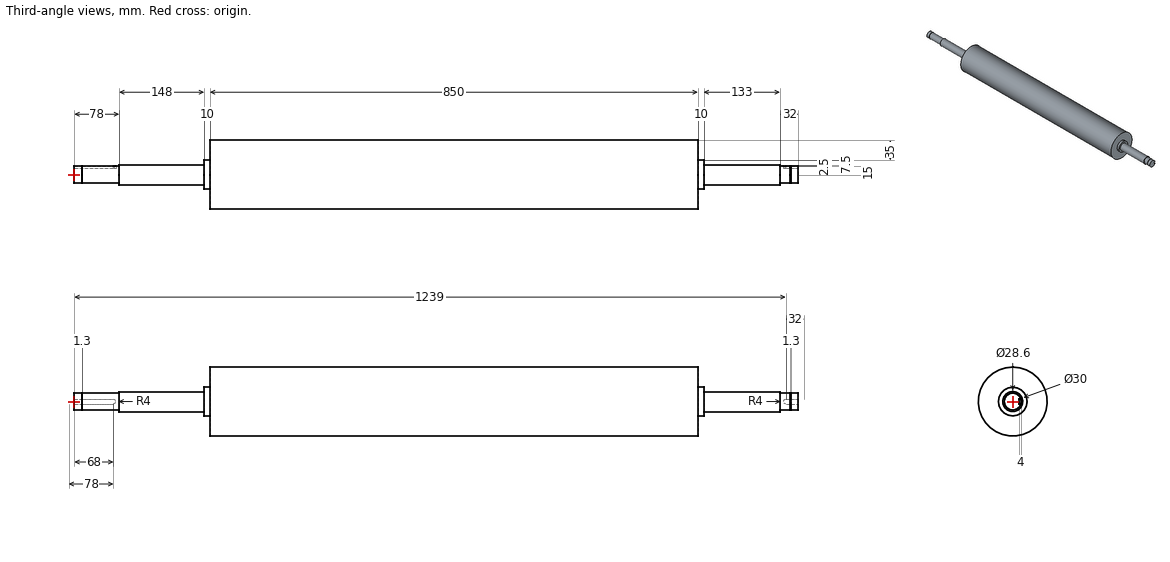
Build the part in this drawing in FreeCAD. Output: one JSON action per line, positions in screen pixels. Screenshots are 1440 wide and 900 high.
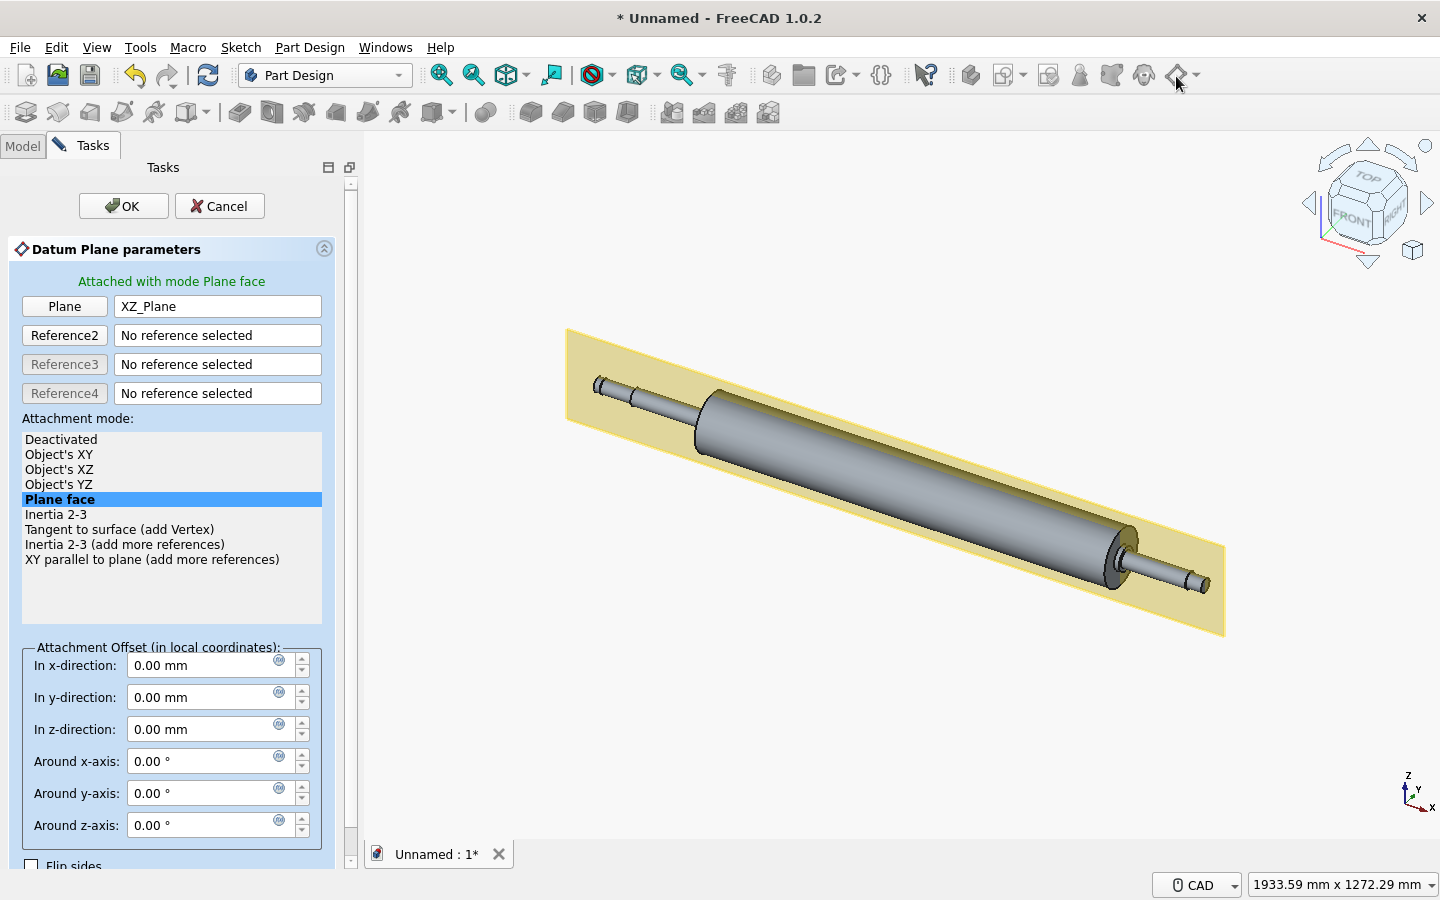
{"action": "triple_click", "coordinate": [210, 729]}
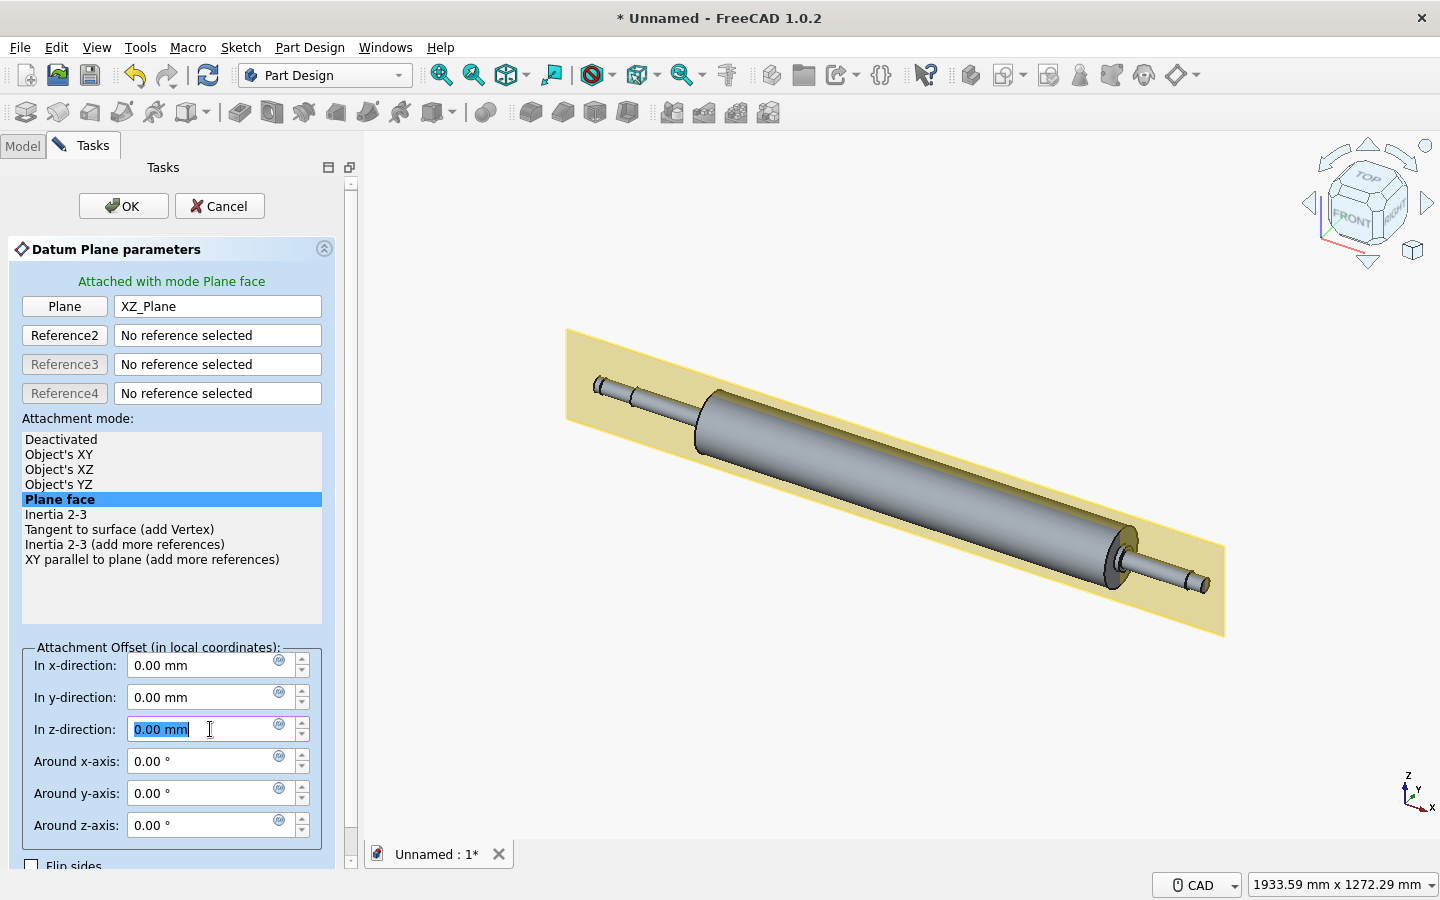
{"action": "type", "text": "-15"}
{"action": "key", "text": "Tab"}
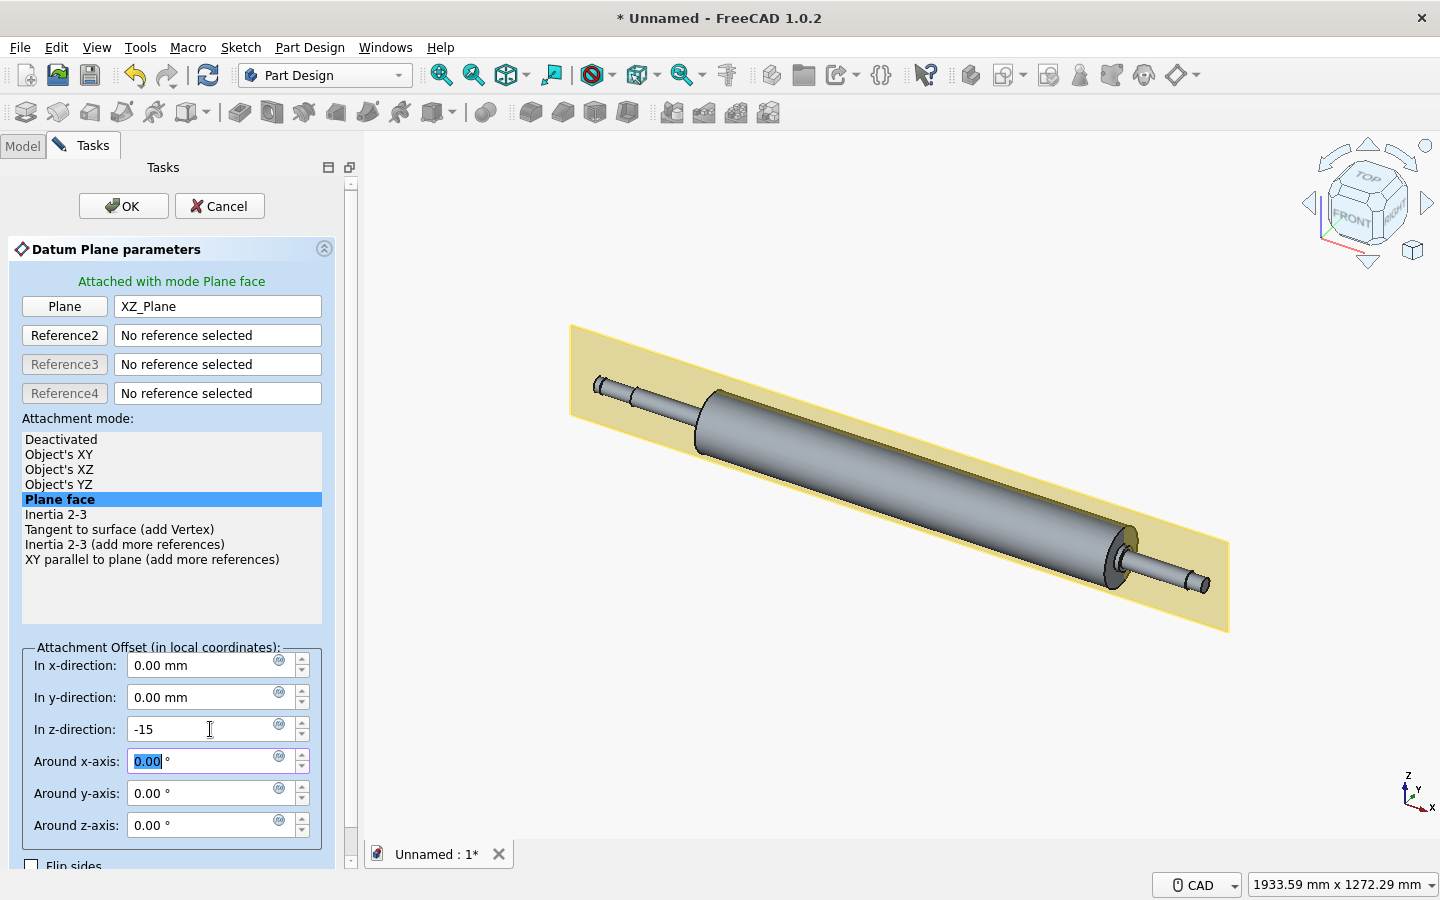
{"action": "left_click", "coordinate": [124, 206]}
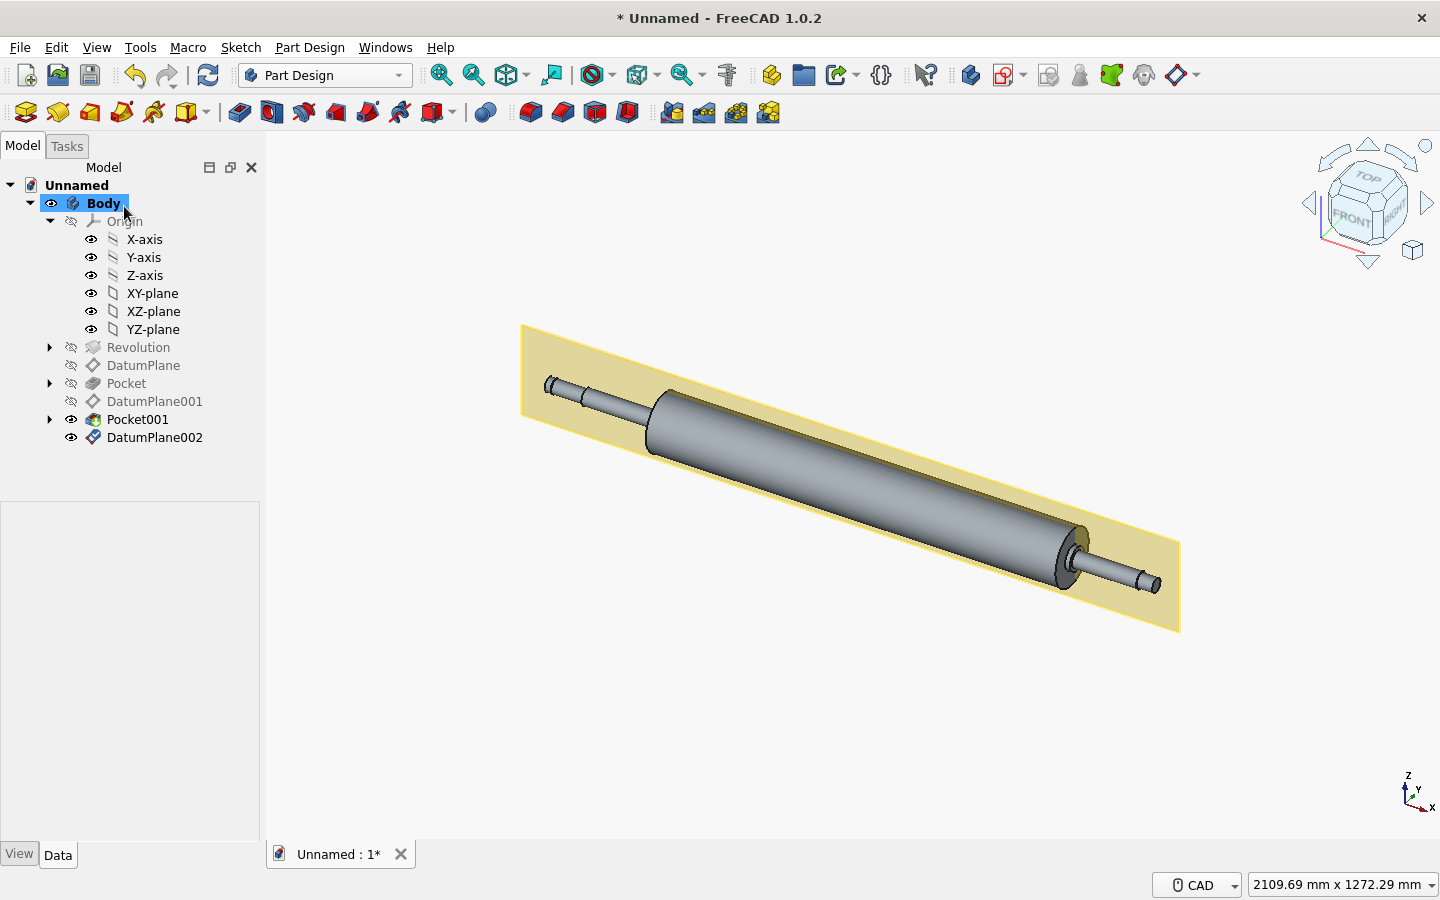
{"action": "left_click", "coordinate": [116, 437]}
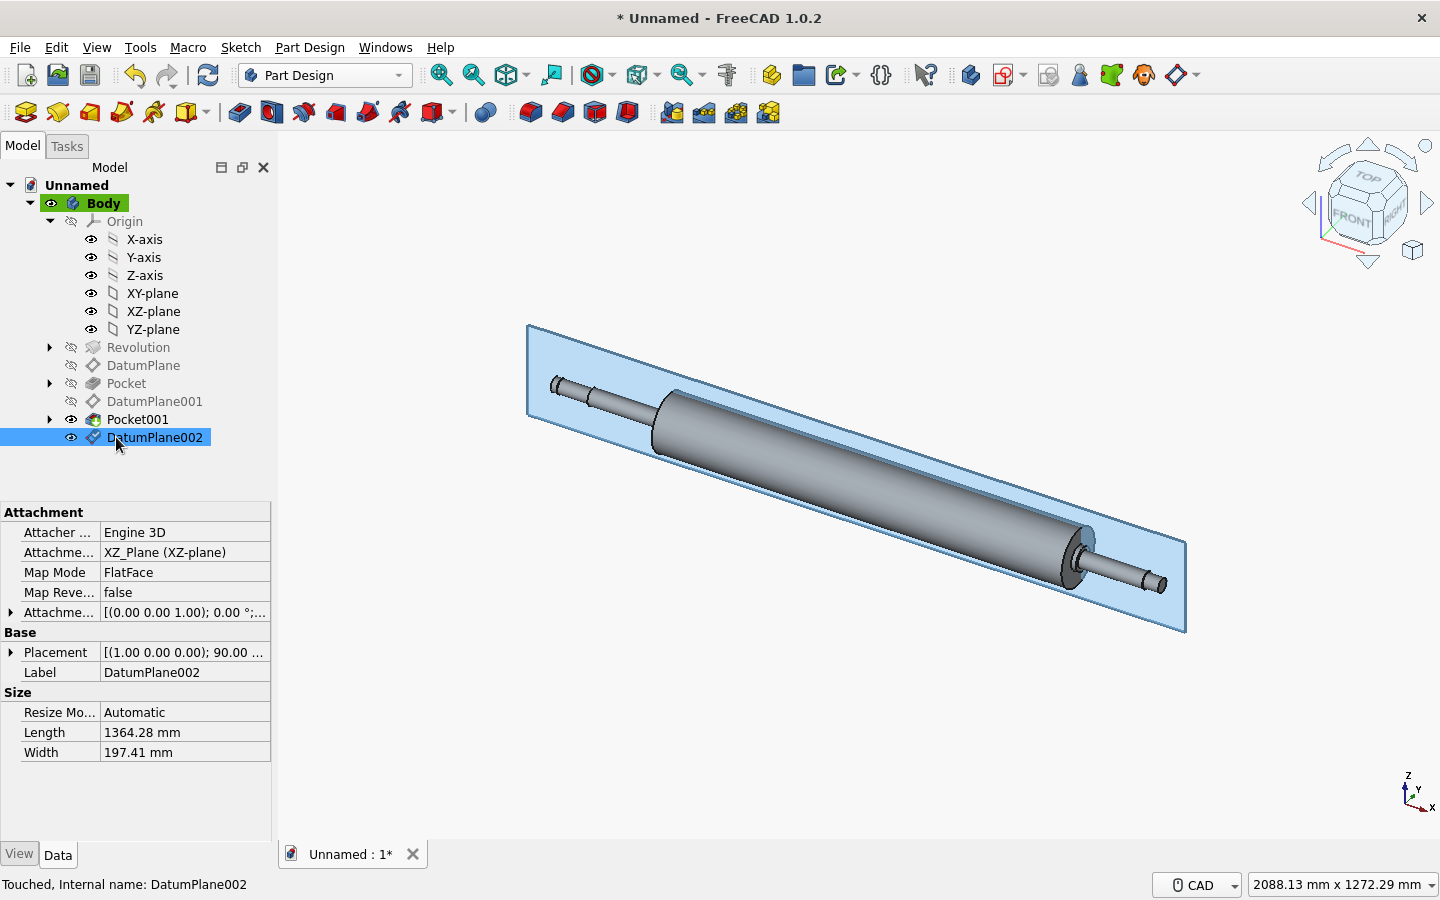
{"action": "left_click", "coordinate": [1004, 76]}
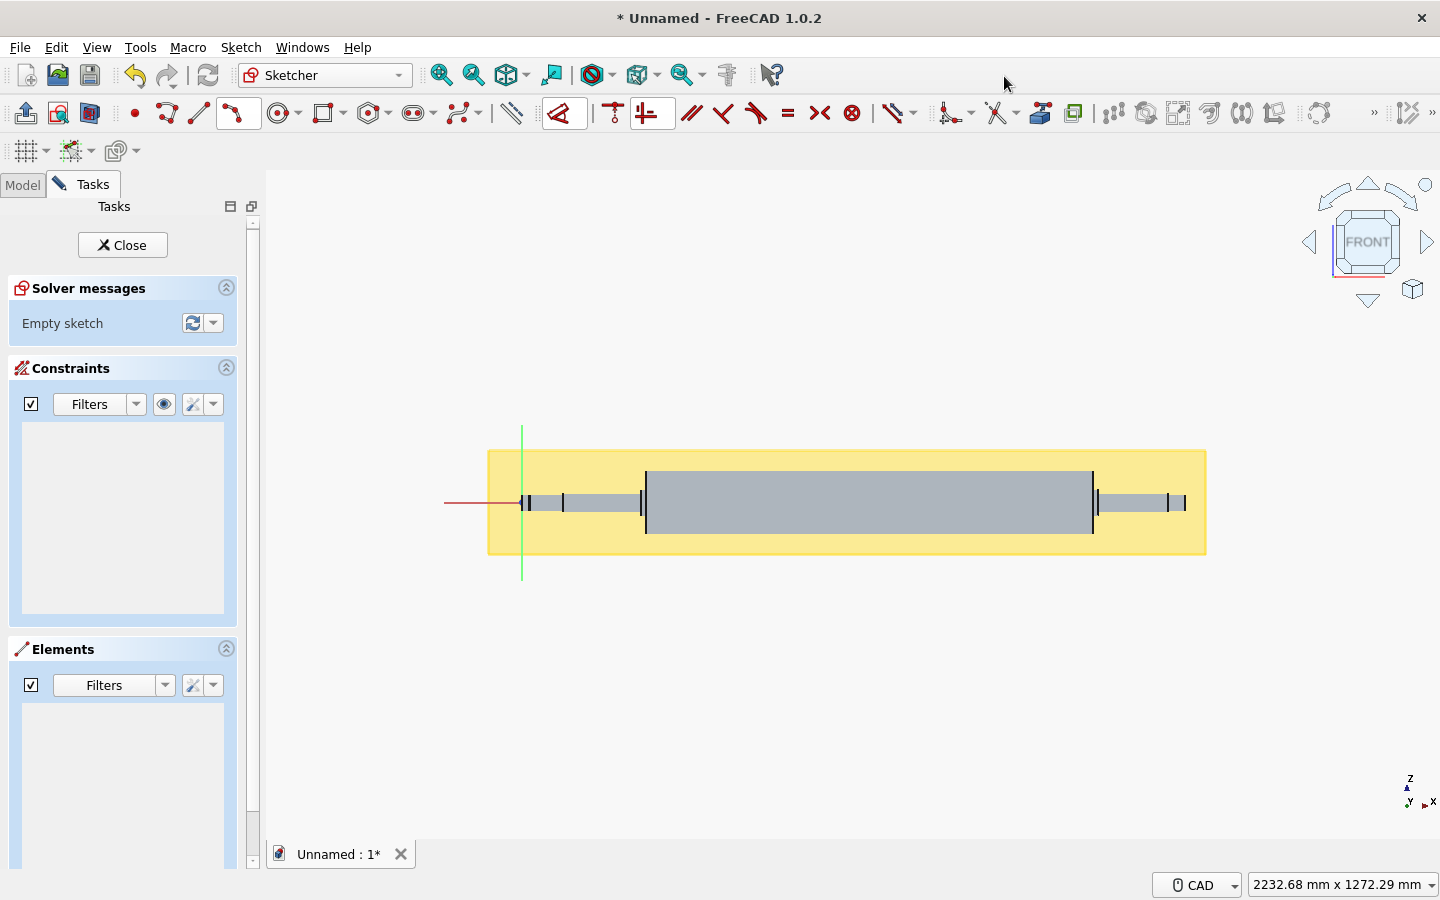
{"action": "key", "text": "q s"}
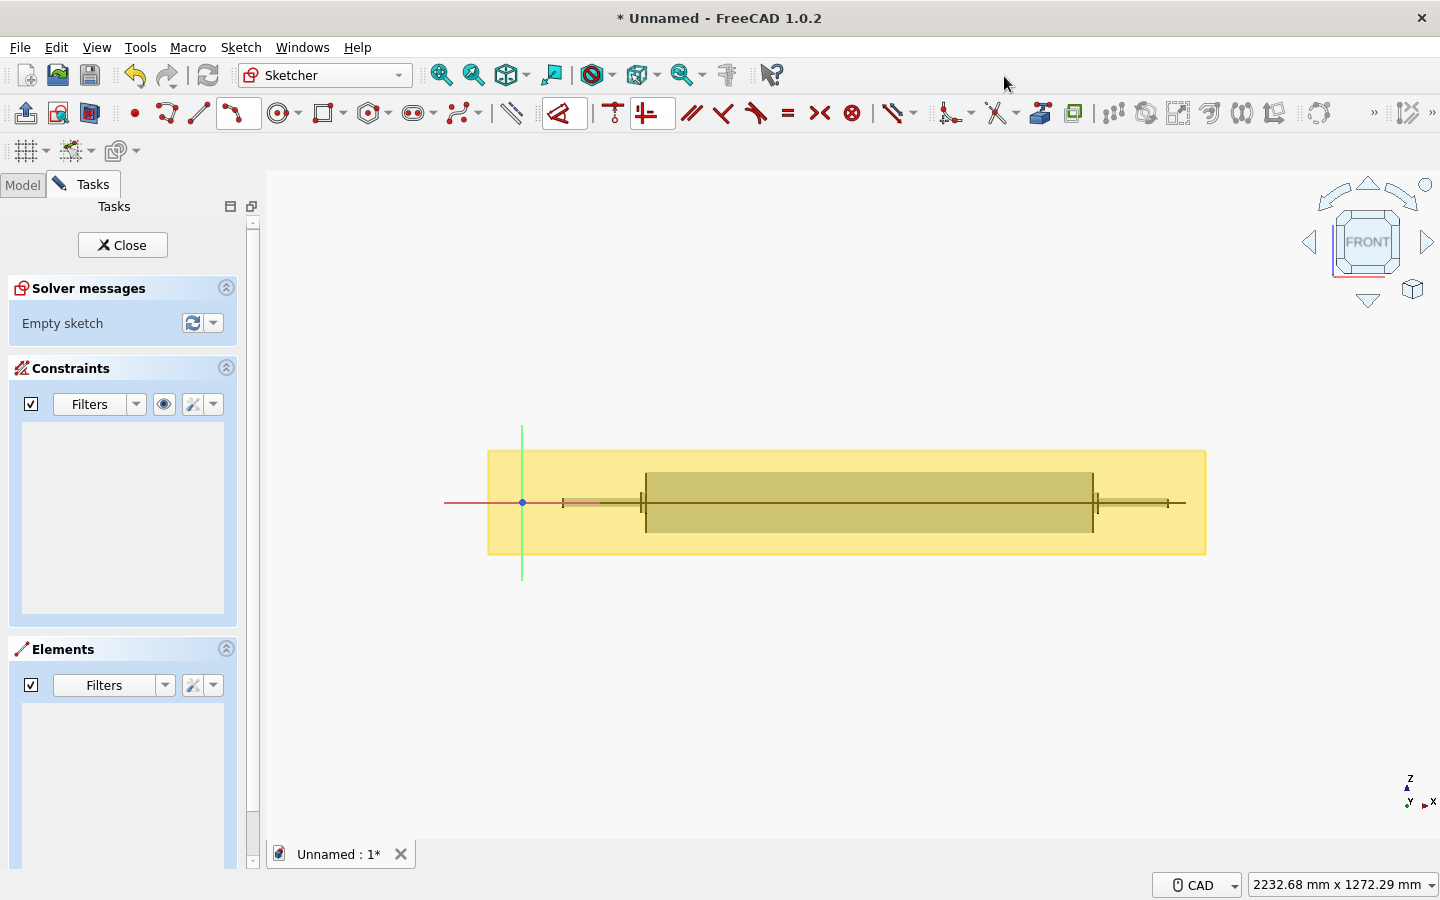
{"action": "scroll", "coordinate": [1202, 503], "scroll_direction": "up", "scroll_amount": 15}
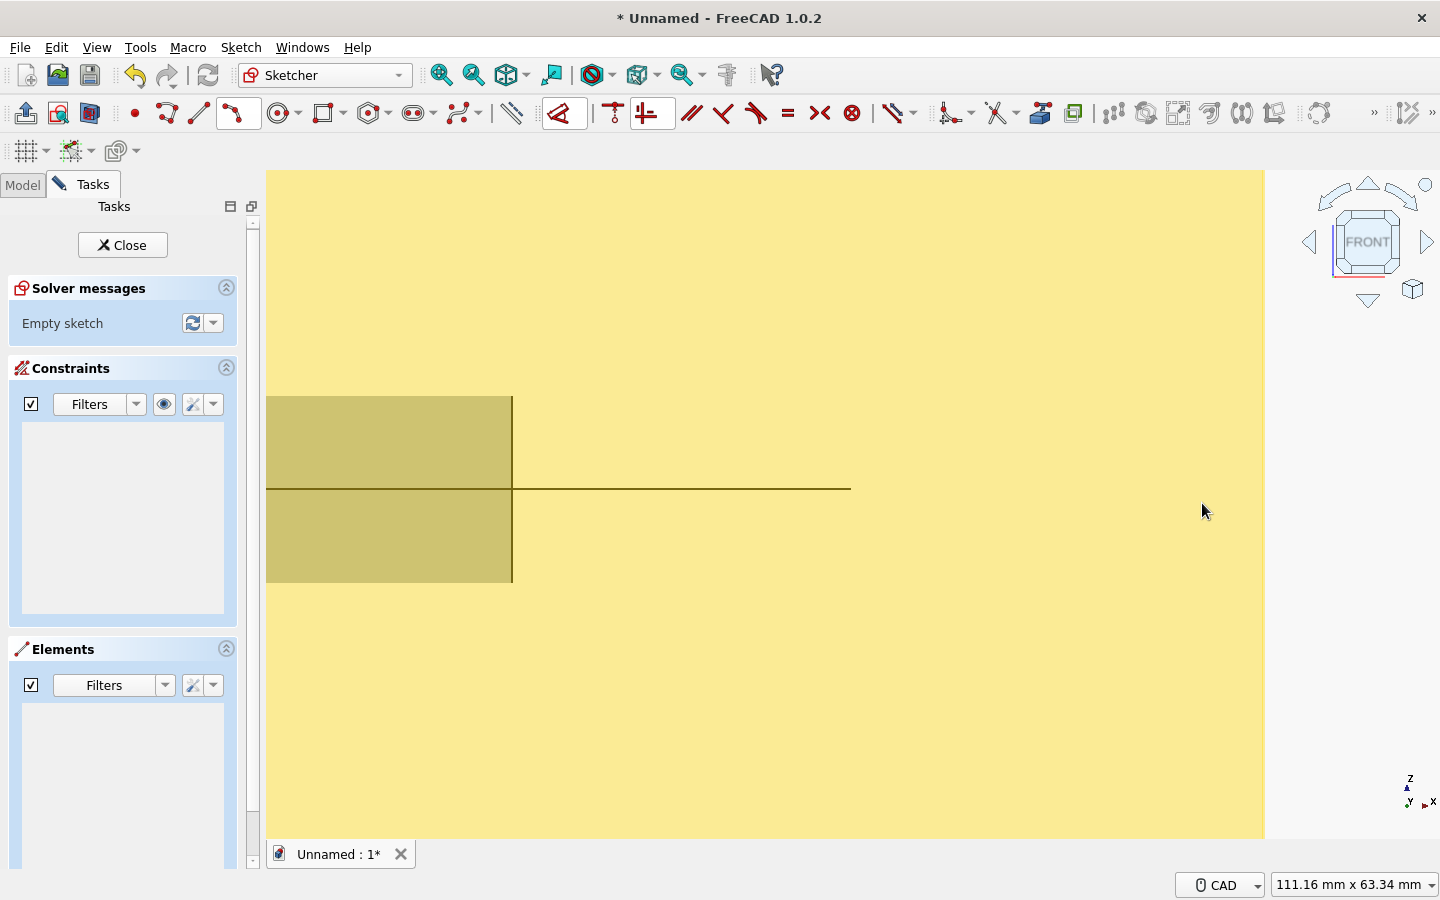
{"action": "scroll", "coordinate": [742, 471], "scroll_direction": "up", "scroll_amount": 3}